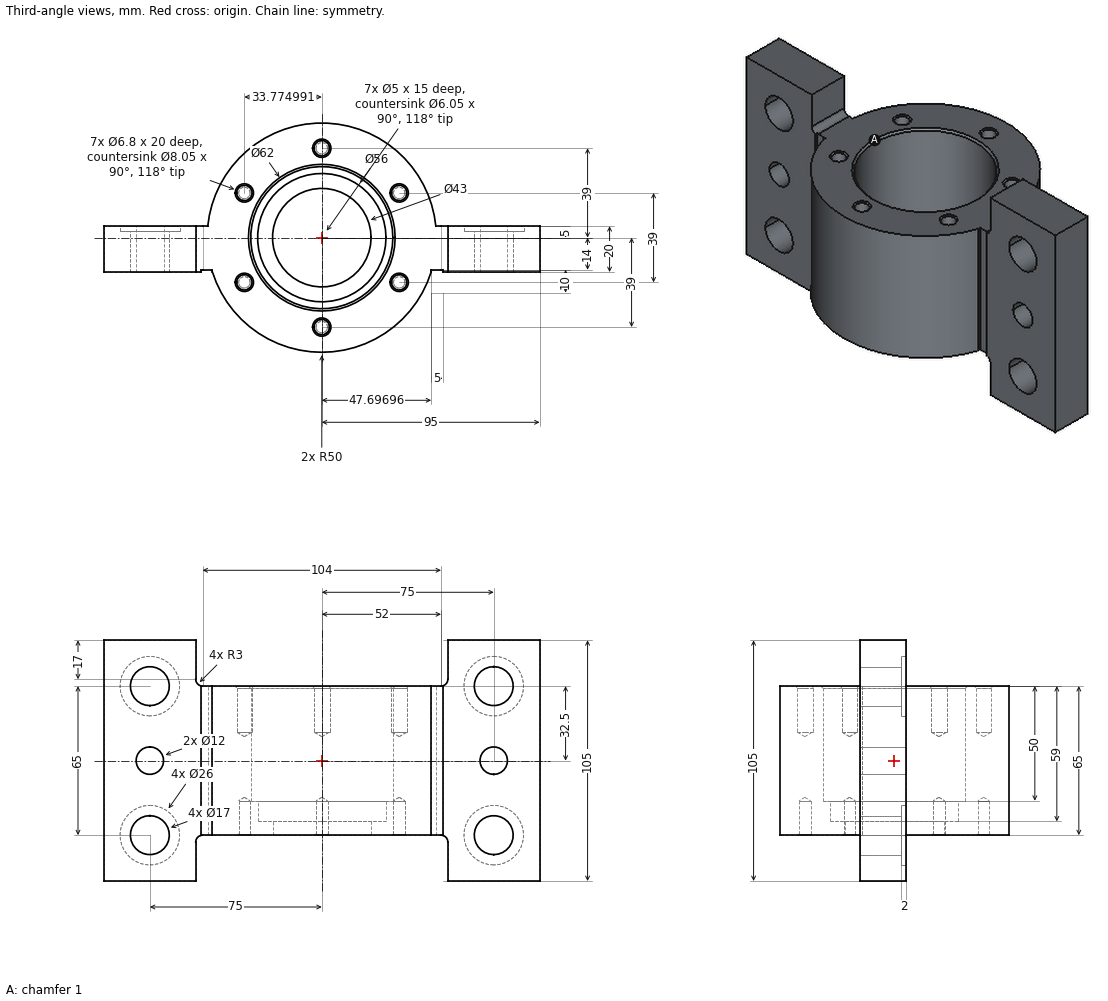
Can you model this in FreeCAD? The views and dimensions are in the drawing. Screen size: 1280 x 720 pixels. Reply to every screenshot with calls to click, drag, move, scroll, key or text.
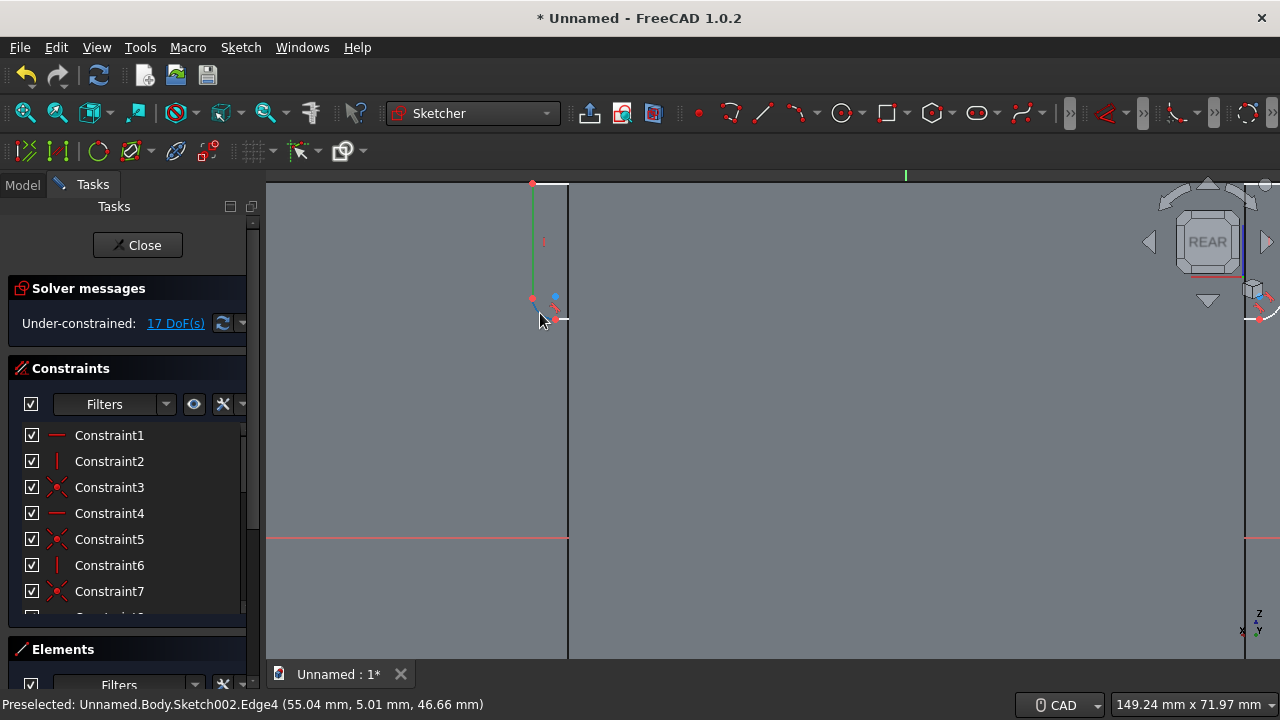
click(540, 313)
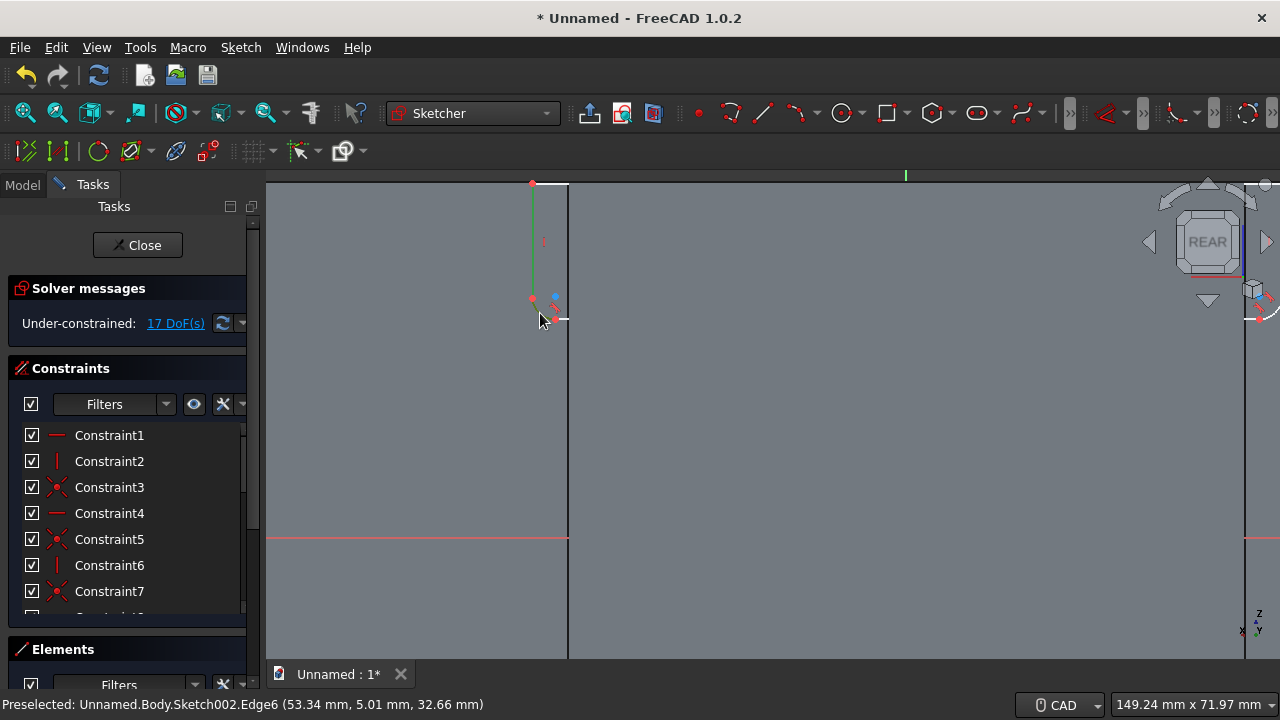
key(t)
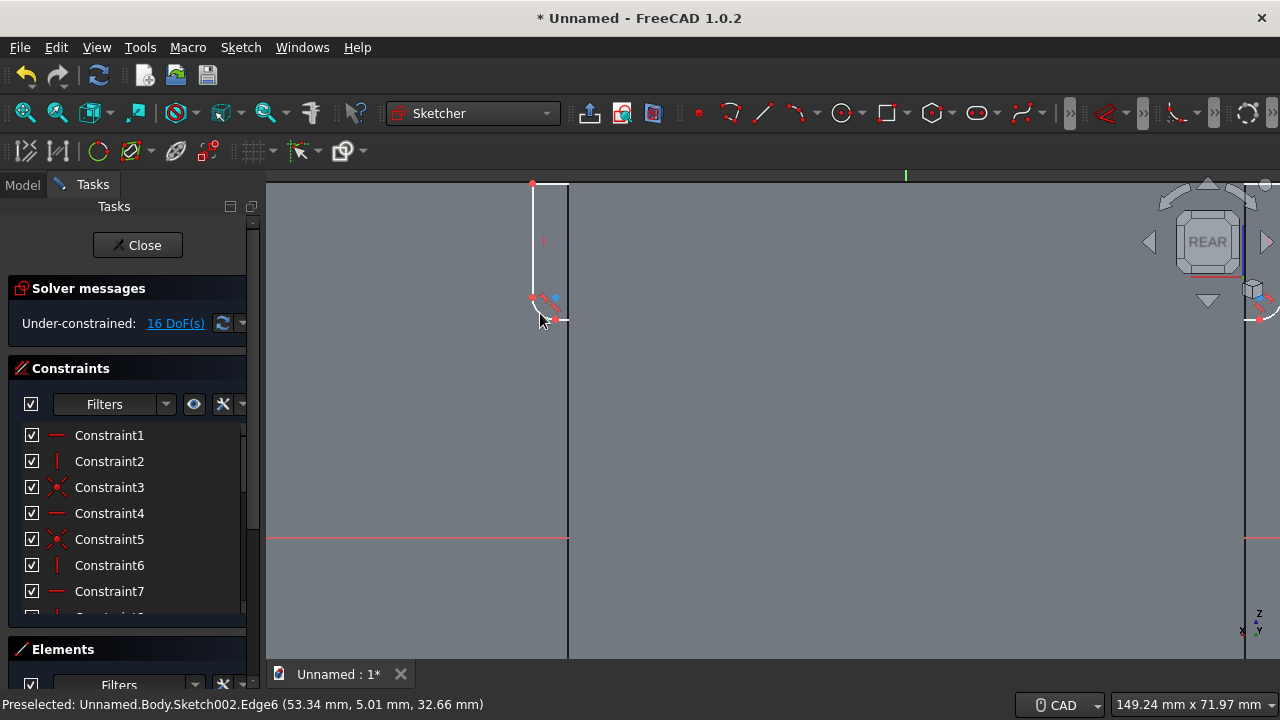
scroll(540, 313, down, 4)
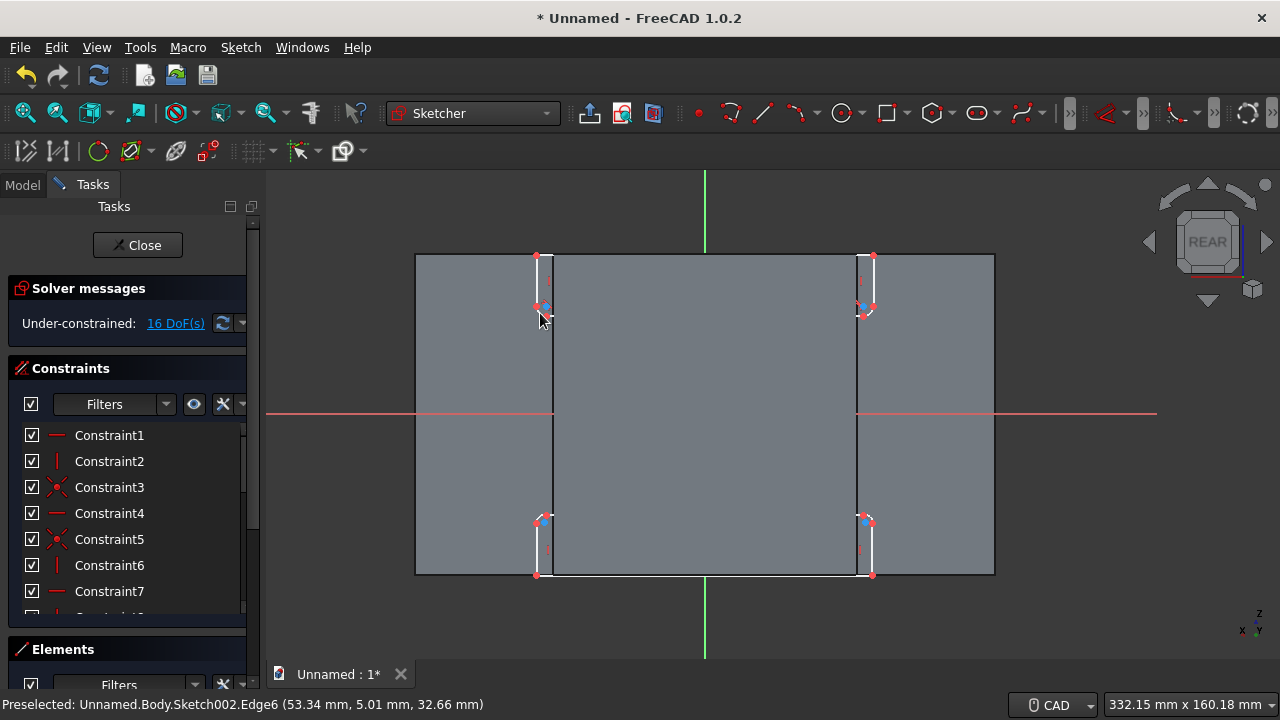
click(768, 515)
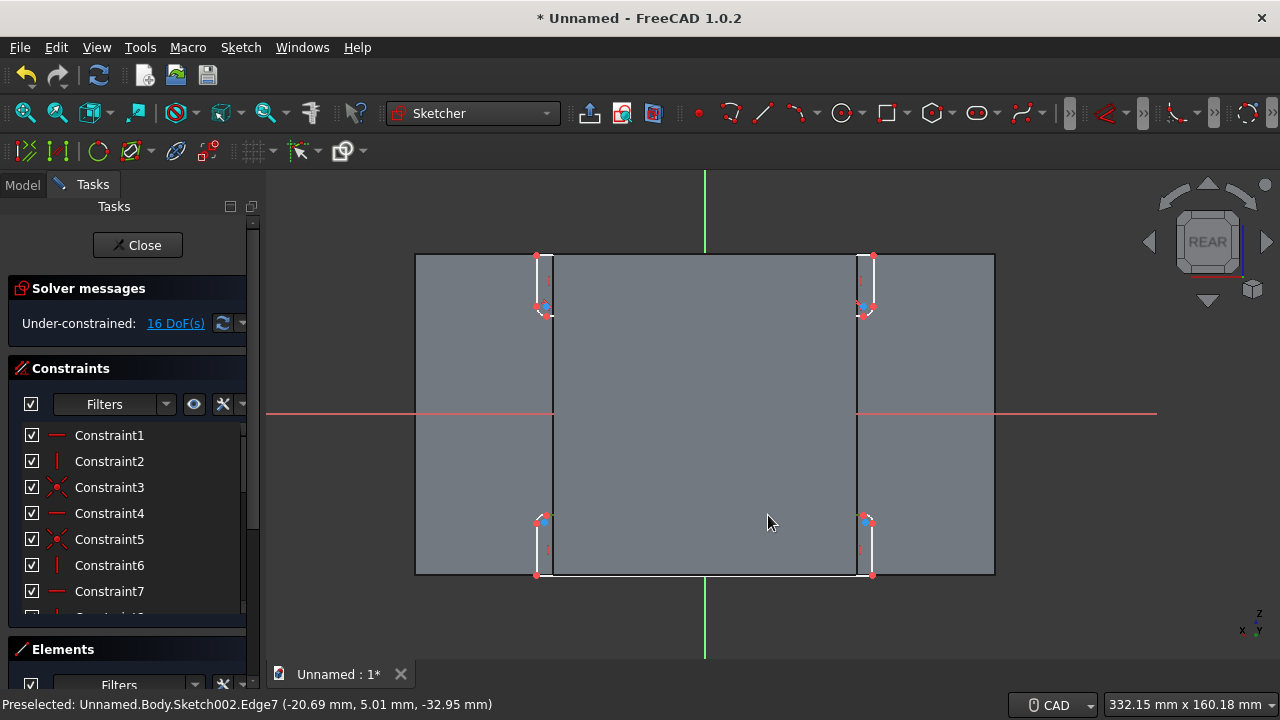
scroll(539, 517, up, 4)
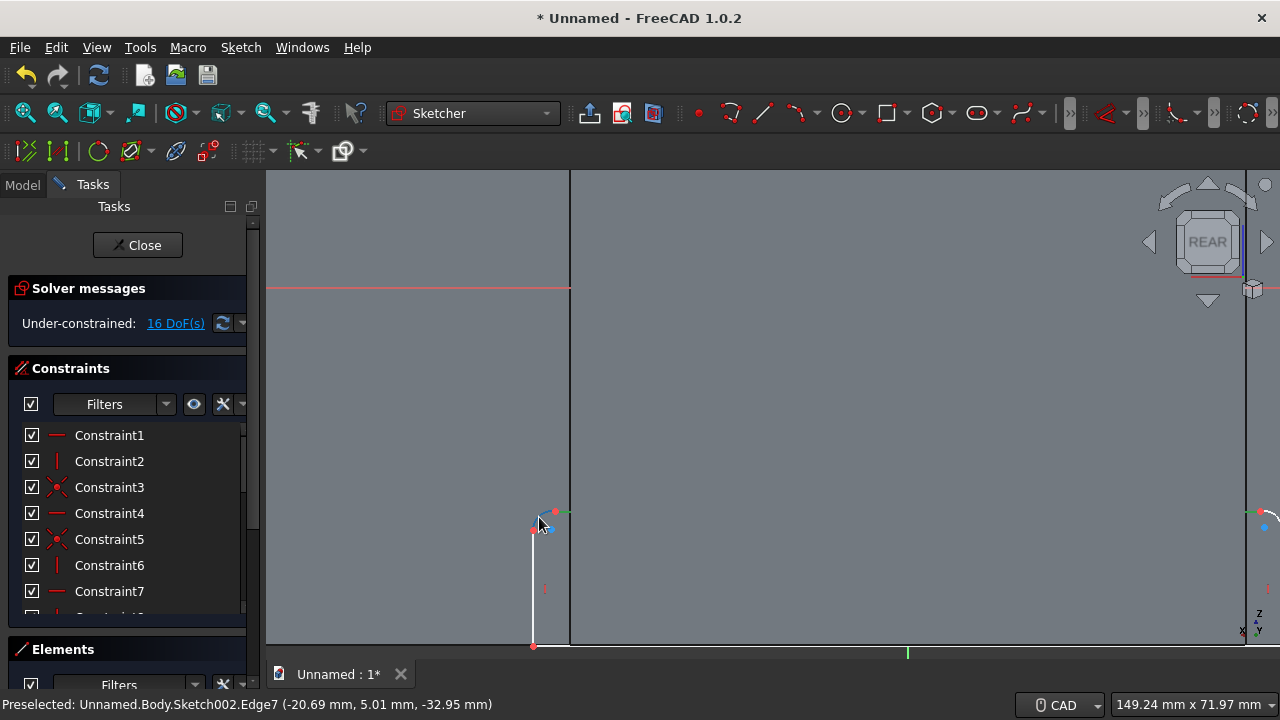
click(540, 515)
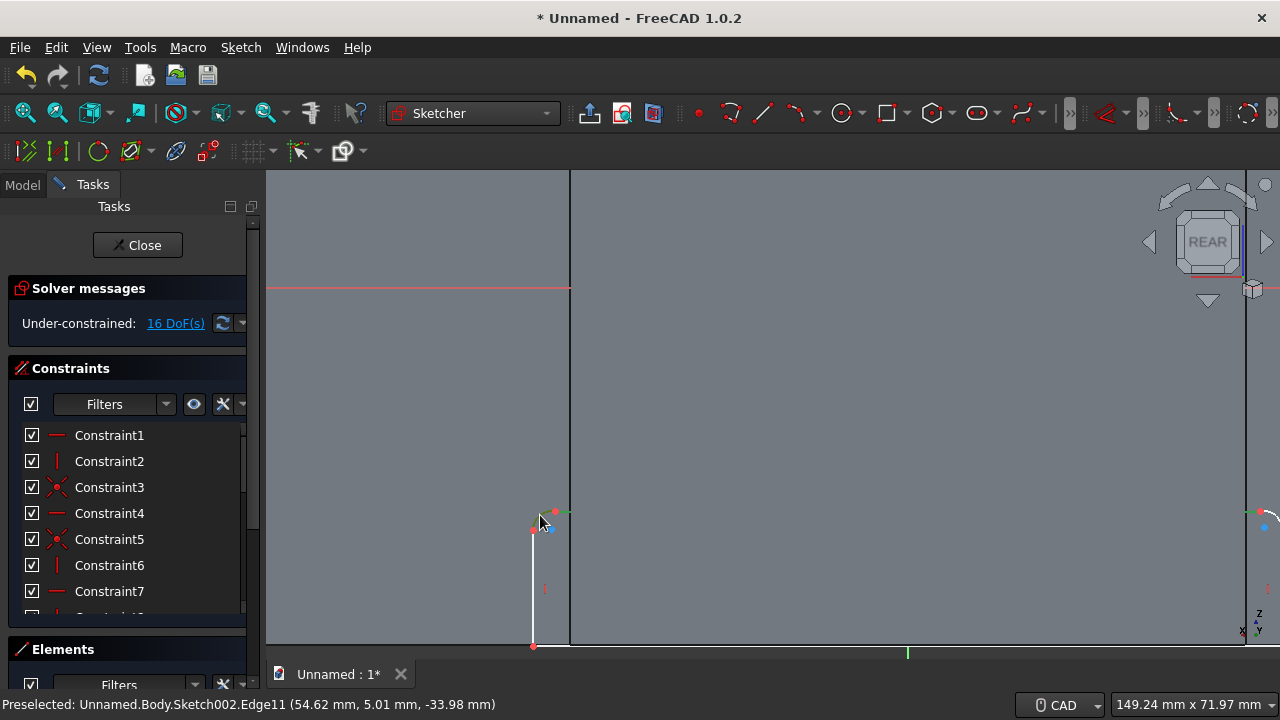
key(t)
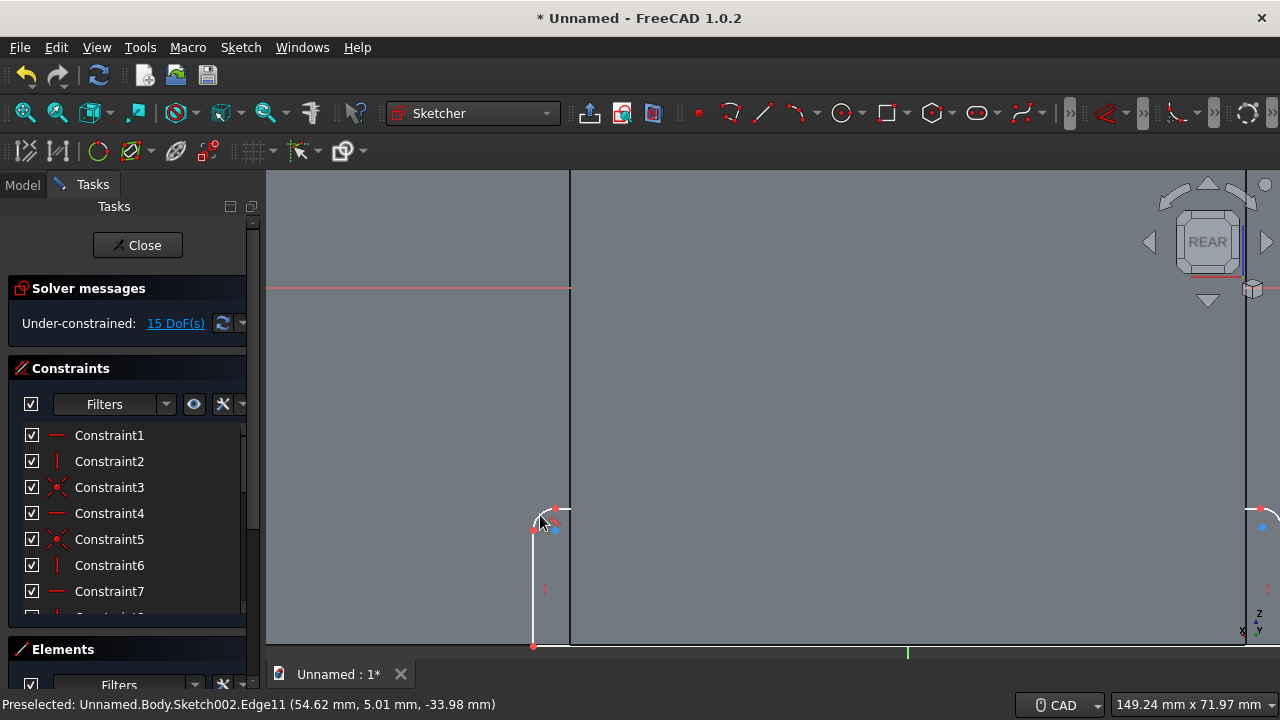
click(1049, 509)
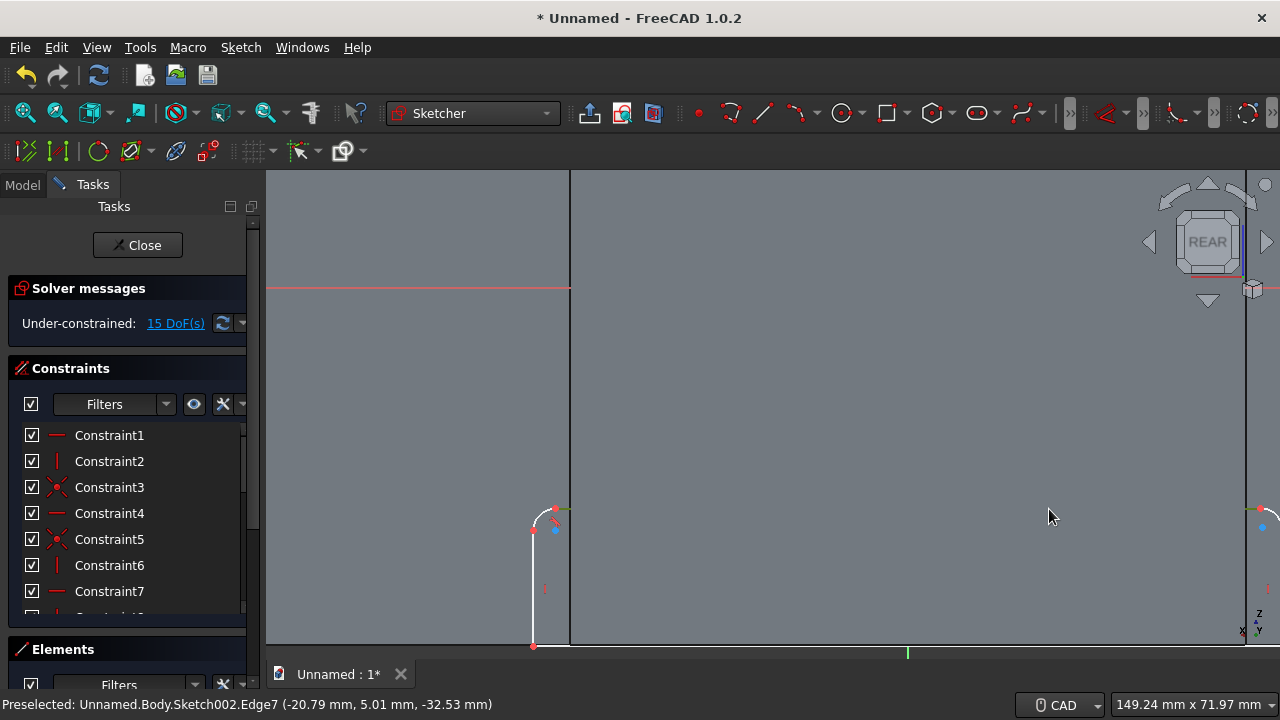
scroll(539, 518, down, 4)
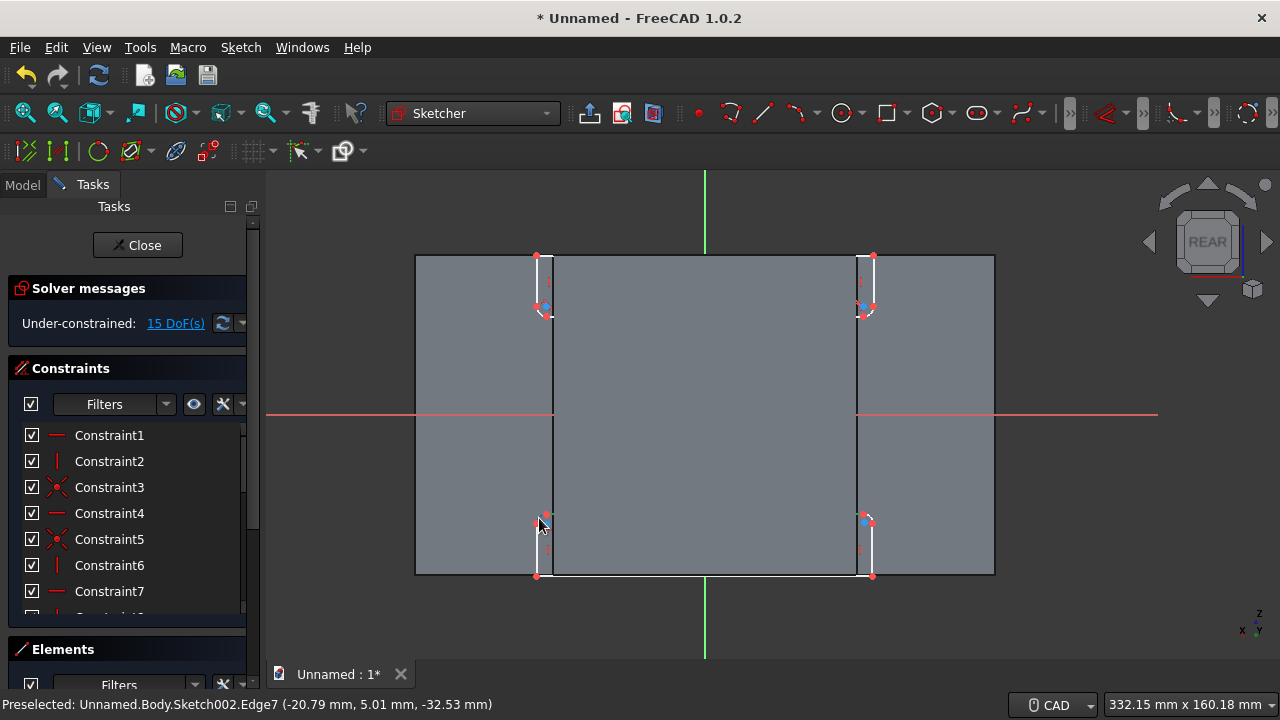
scroll(872, 519, up, 6)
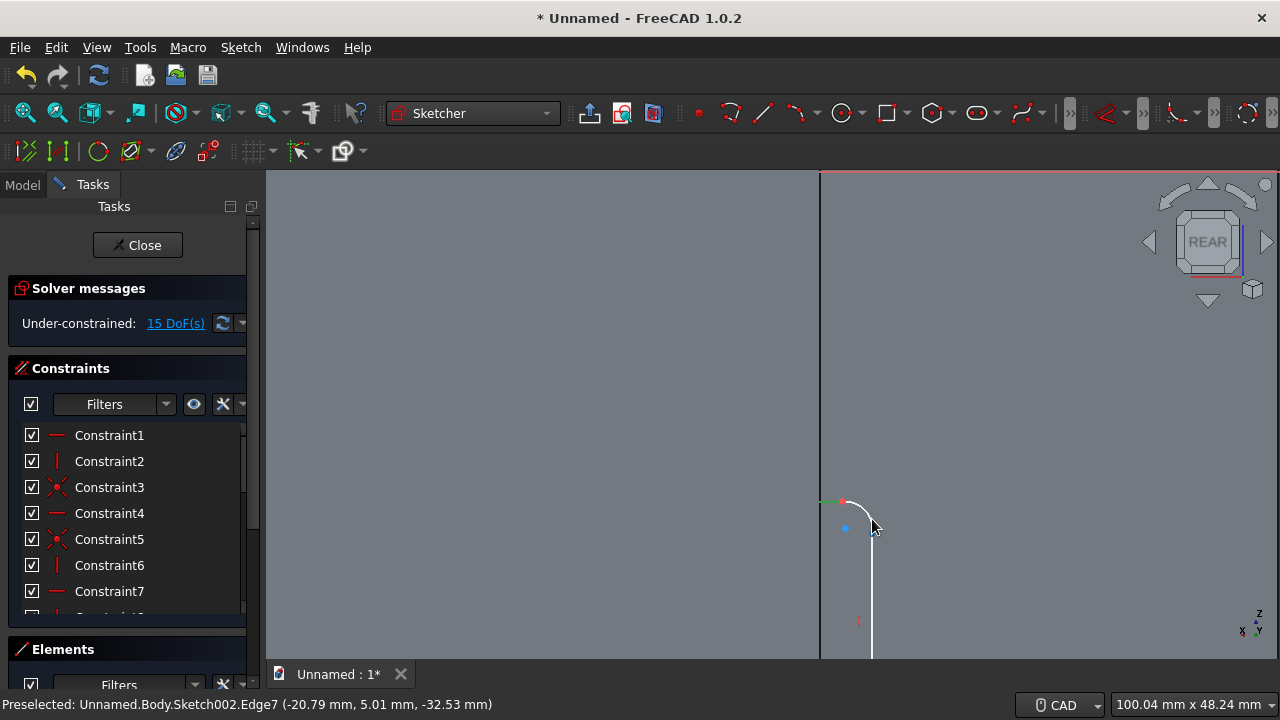
click(870, 519)